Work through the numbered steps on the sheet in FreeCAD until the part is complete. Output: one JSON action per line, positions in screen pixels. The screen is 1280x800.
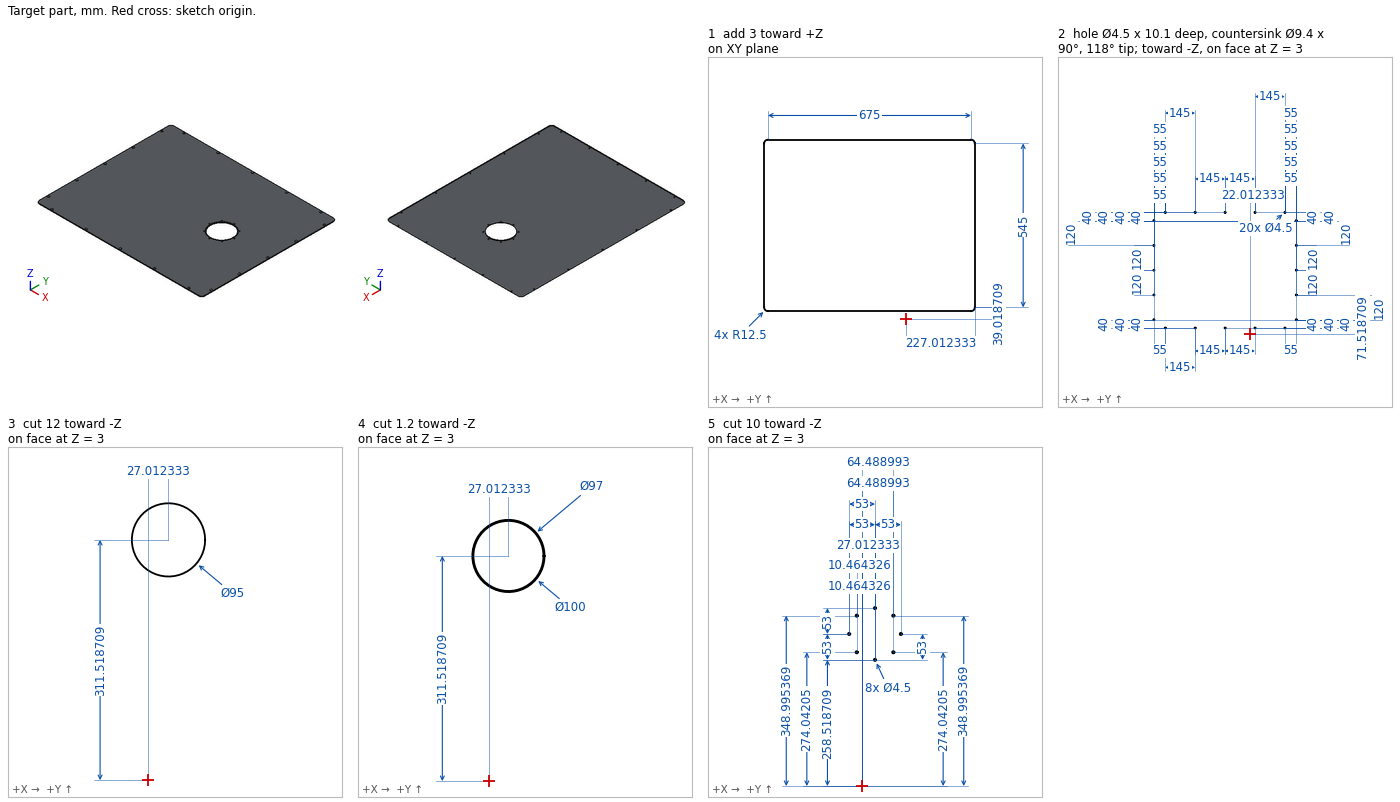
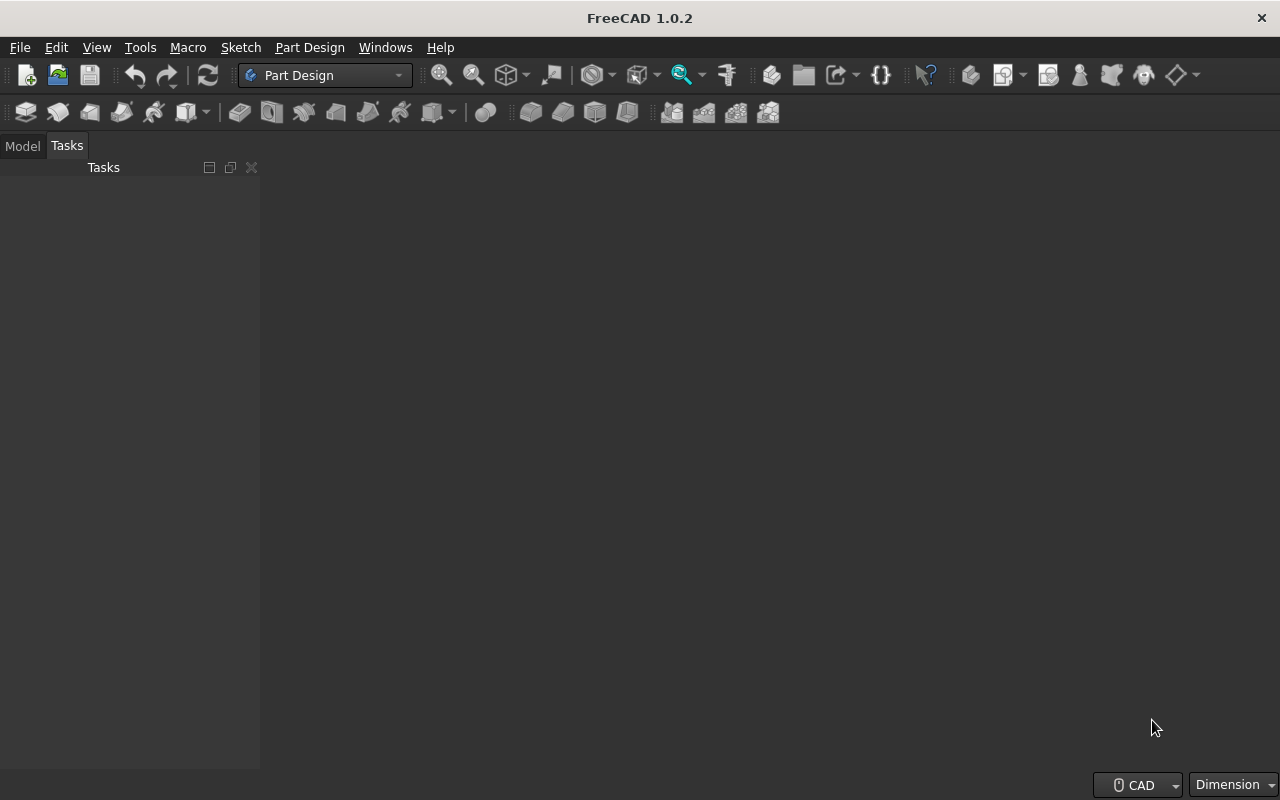
{"action": "left_click", "coordinate": [26, 76]}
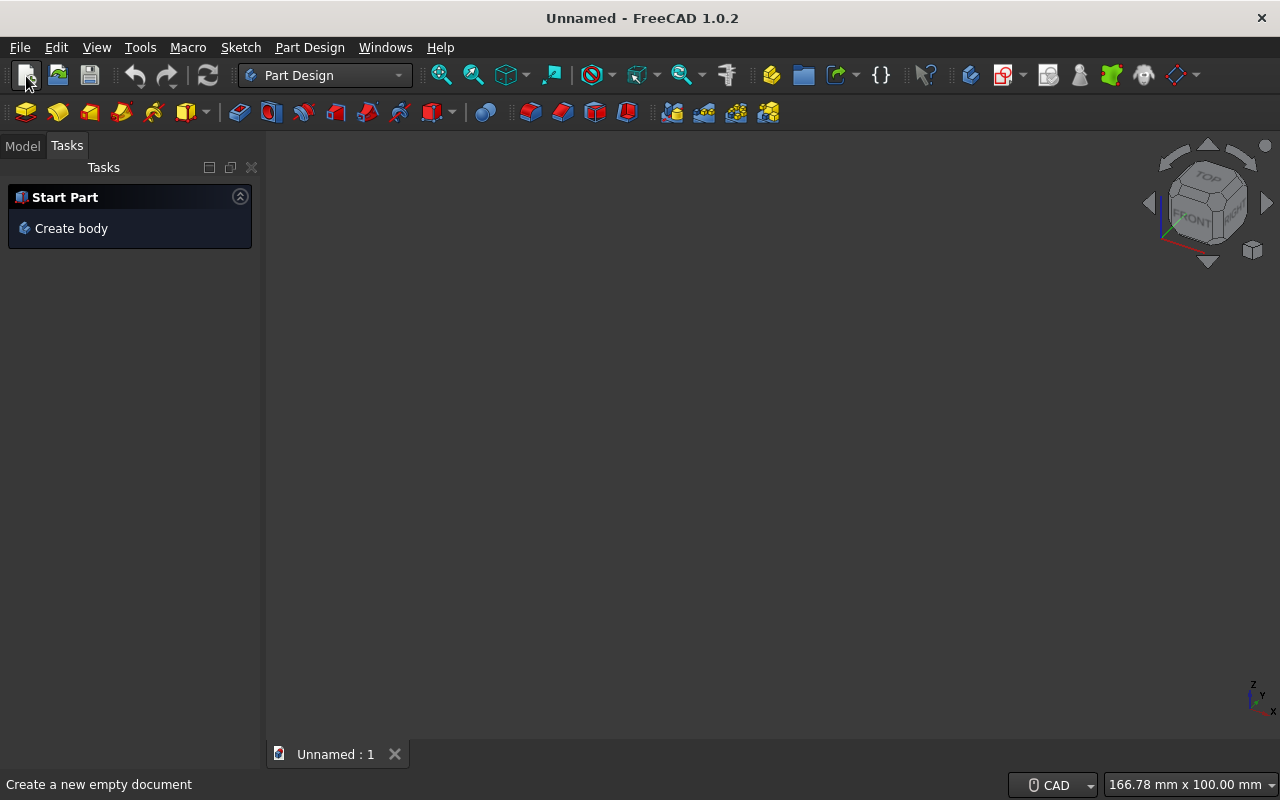
{"action": "left_click", "coordinate": [1004, 76]}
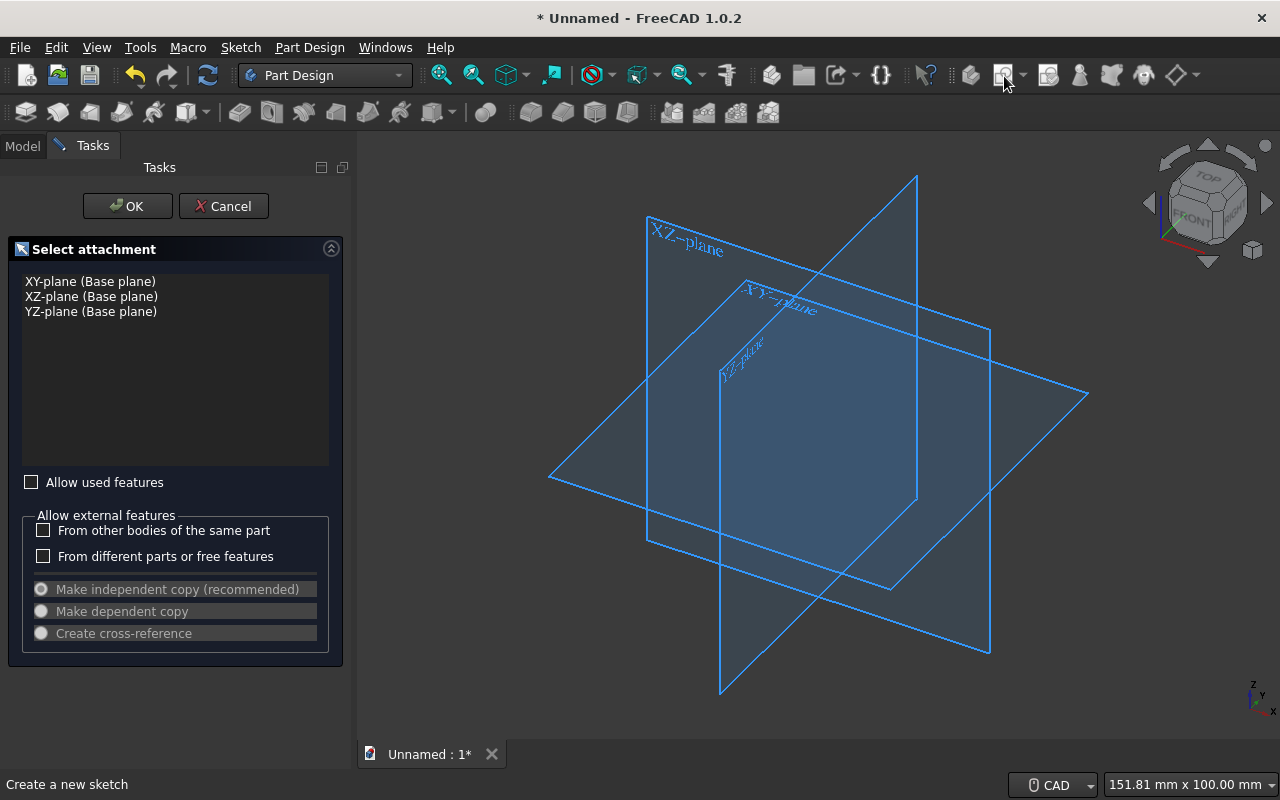
{"action": "left_click", "coordinate": [82, 282]}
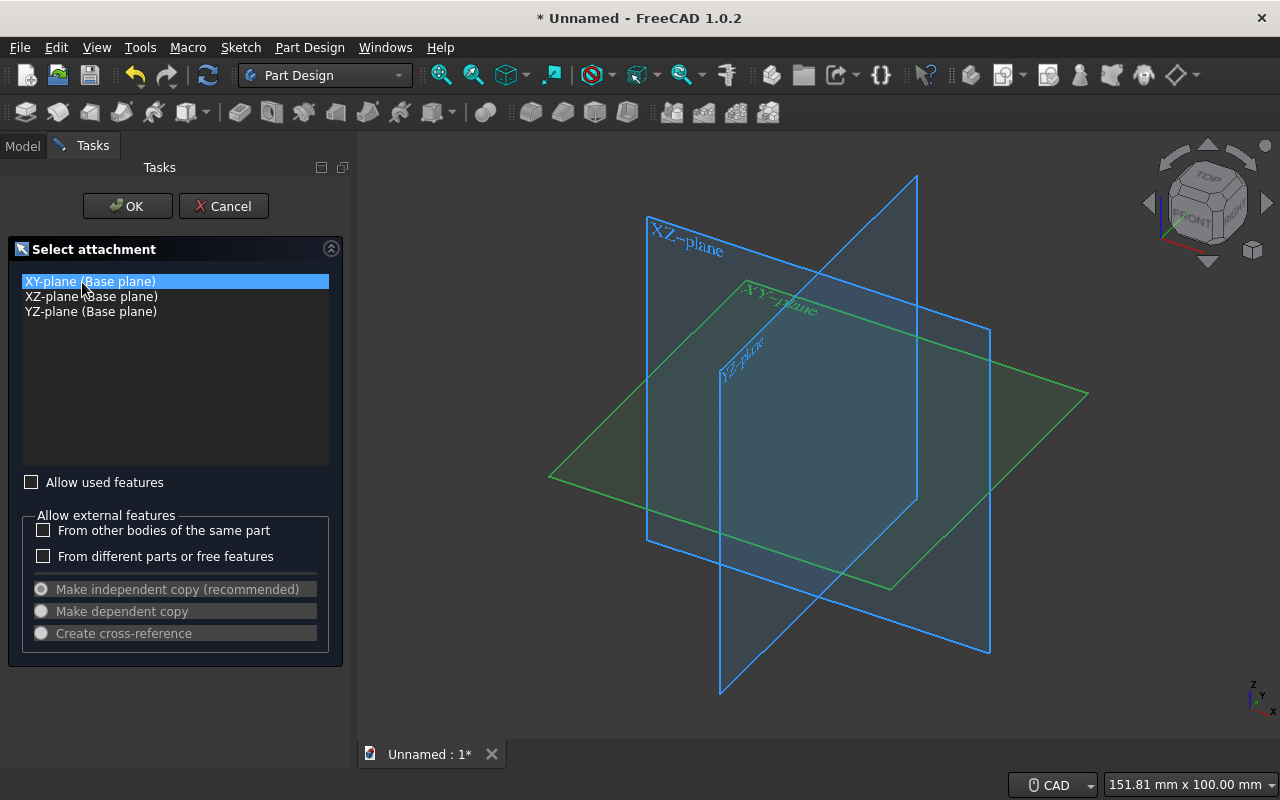
{"action": "left_click", "coordinate": [128, 206]}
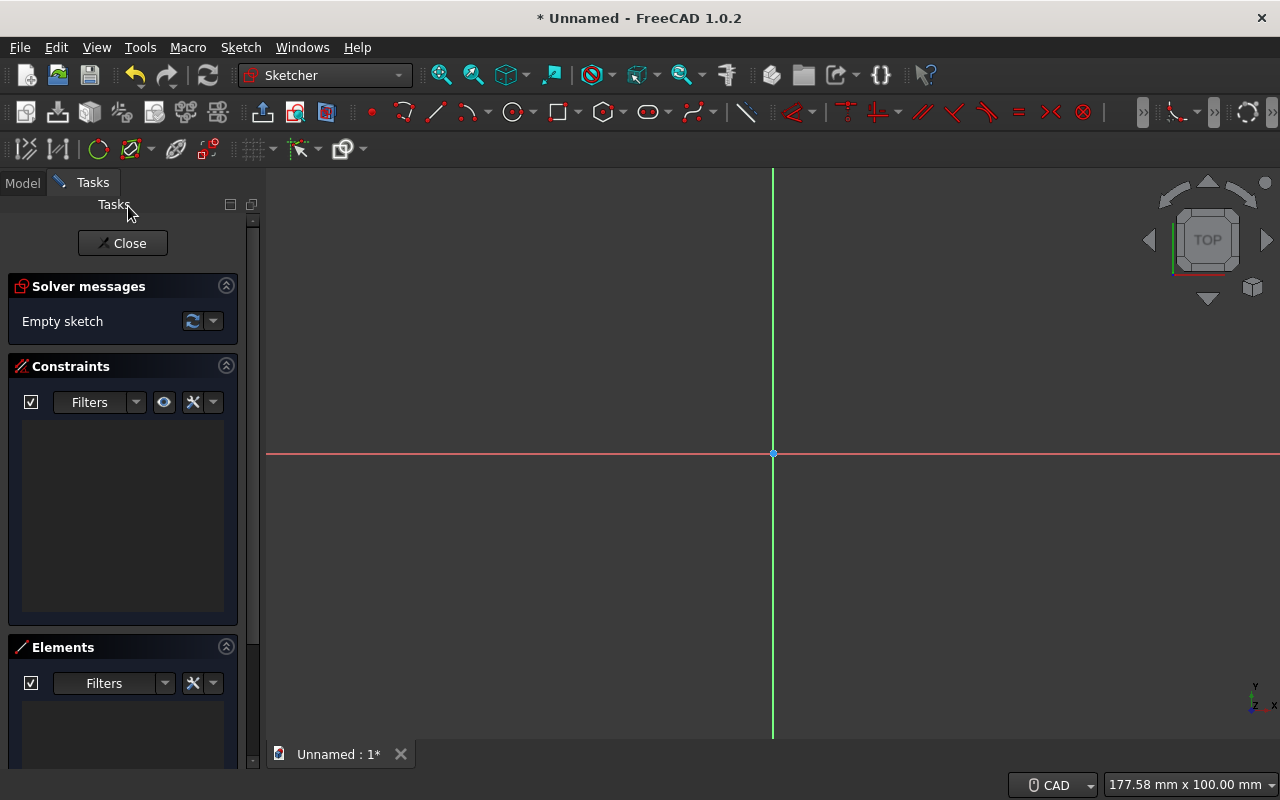
{"action": "scroll", "coordinate": [783, 666], "scroll_direction": "down", "scroll_amount": 11}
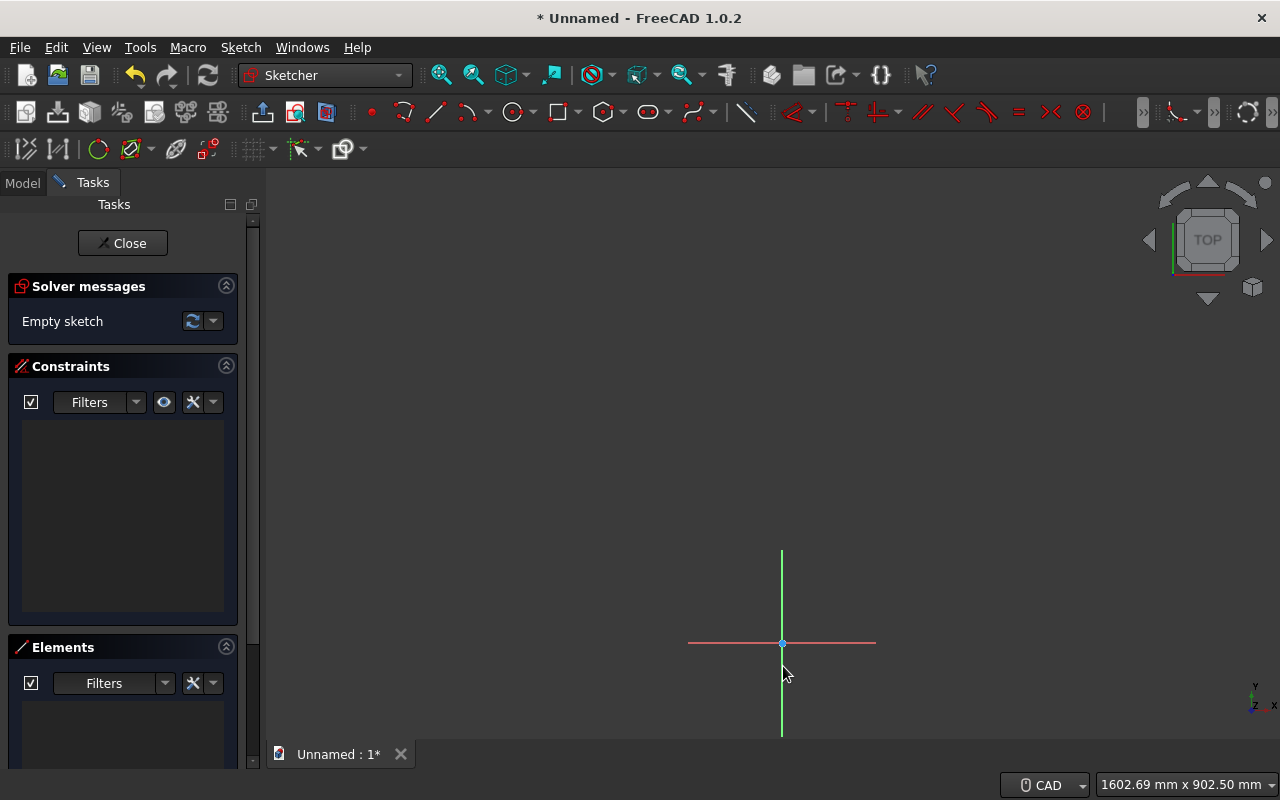
{"action": "left_click", "coordinate": [436, 112]}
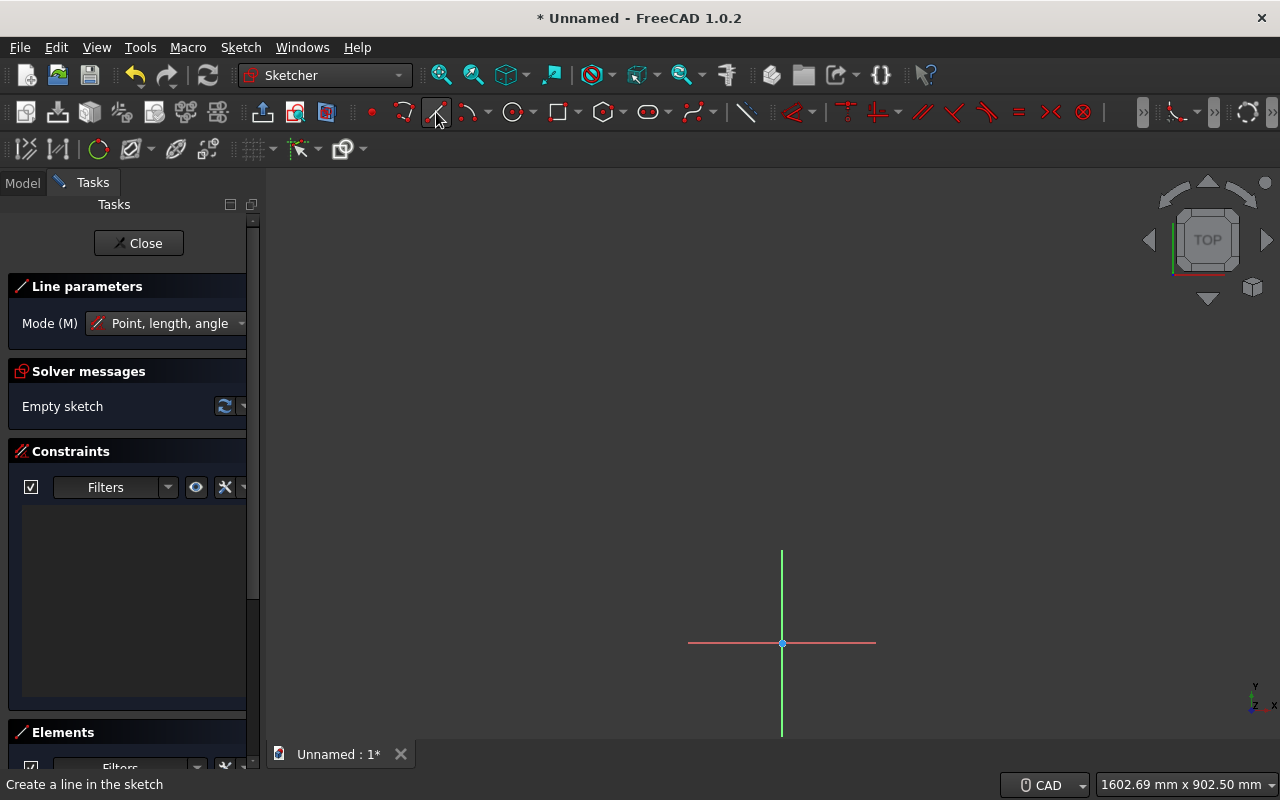
{"action": "left_click", "coordinate": [926, 619]}
{"action": "left_click", "coordinate": [926, 274]}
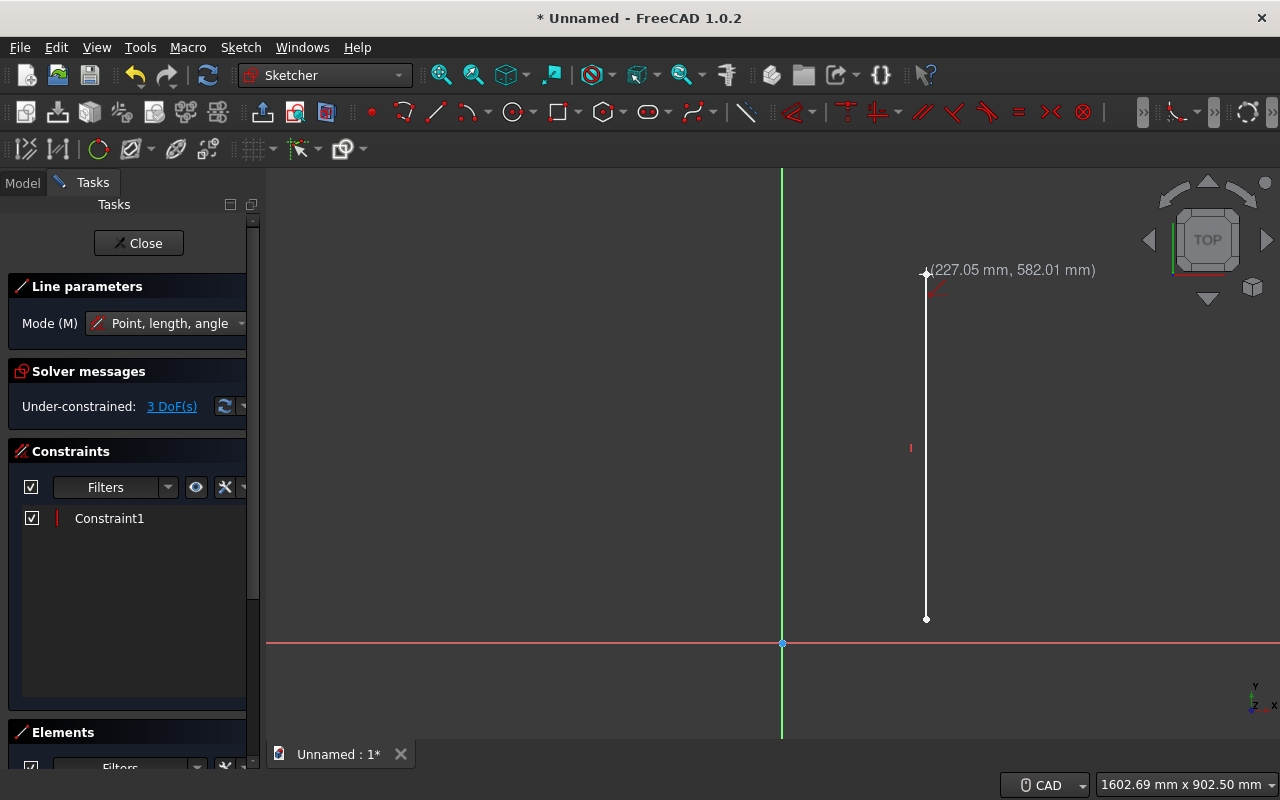
{"action": "scroll", "coordinate": [918, 266], "scroll_direction": "up", "scroll_amount": 2}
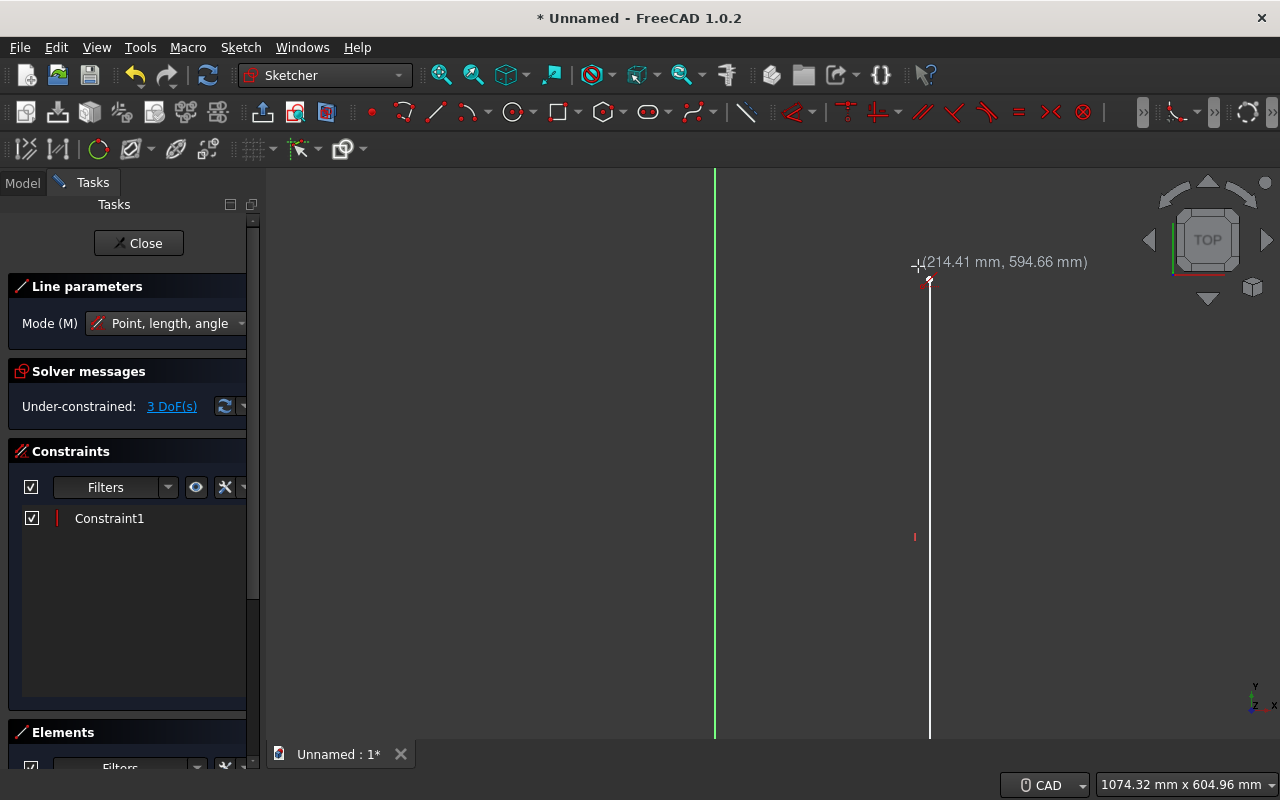
{"action": "left_click", "coordinate": [918, 266]}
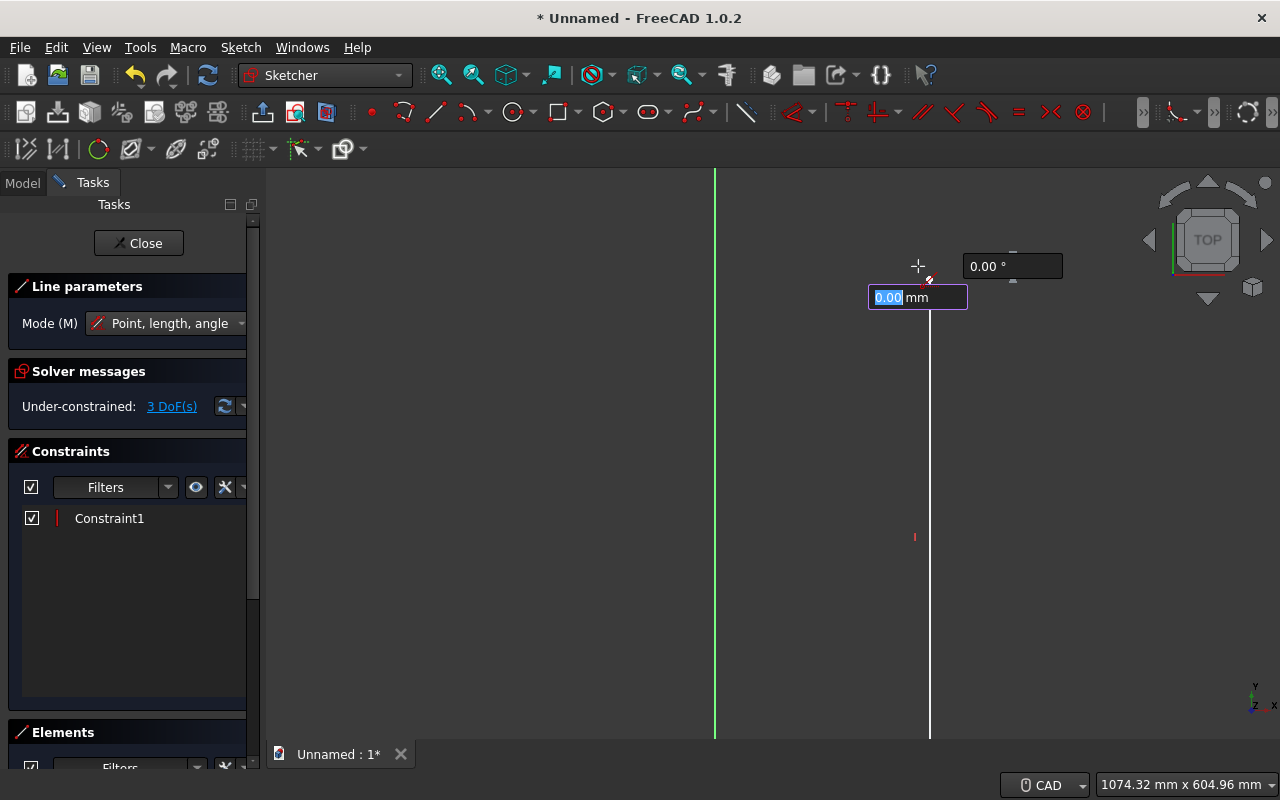
{"action": "scroll", "coordinate": [919, 263], "scroll_direction": "down", "scroll_amount": 2}